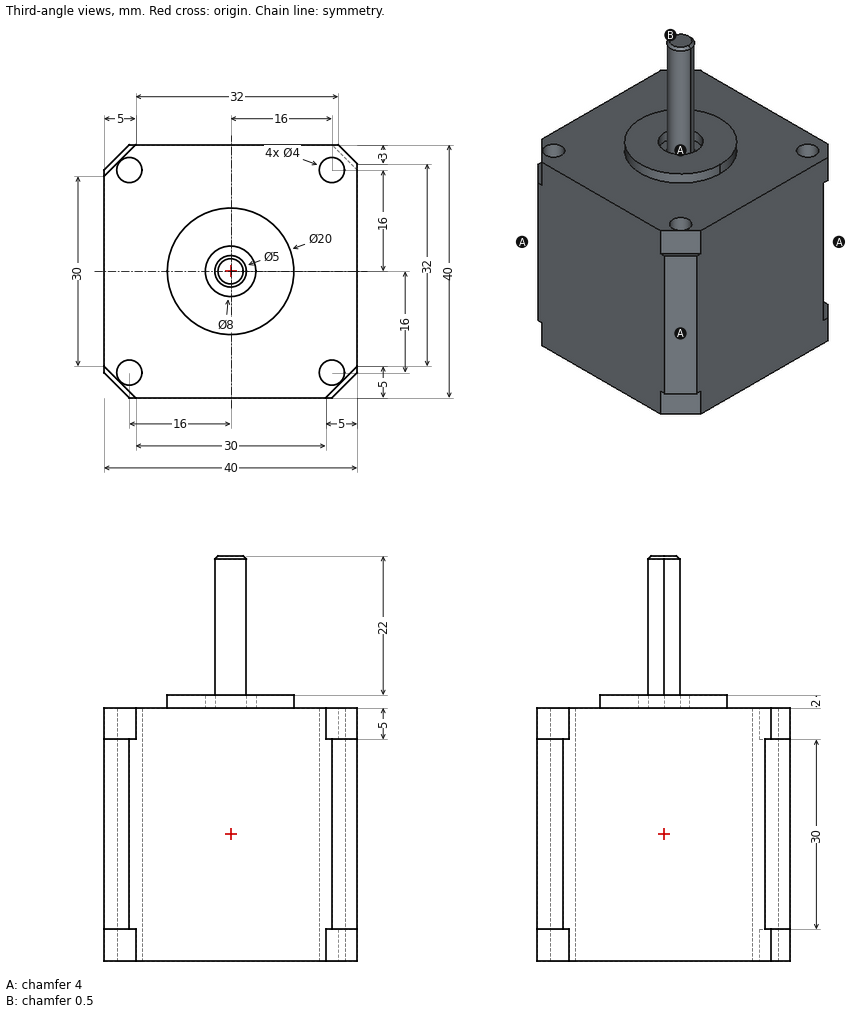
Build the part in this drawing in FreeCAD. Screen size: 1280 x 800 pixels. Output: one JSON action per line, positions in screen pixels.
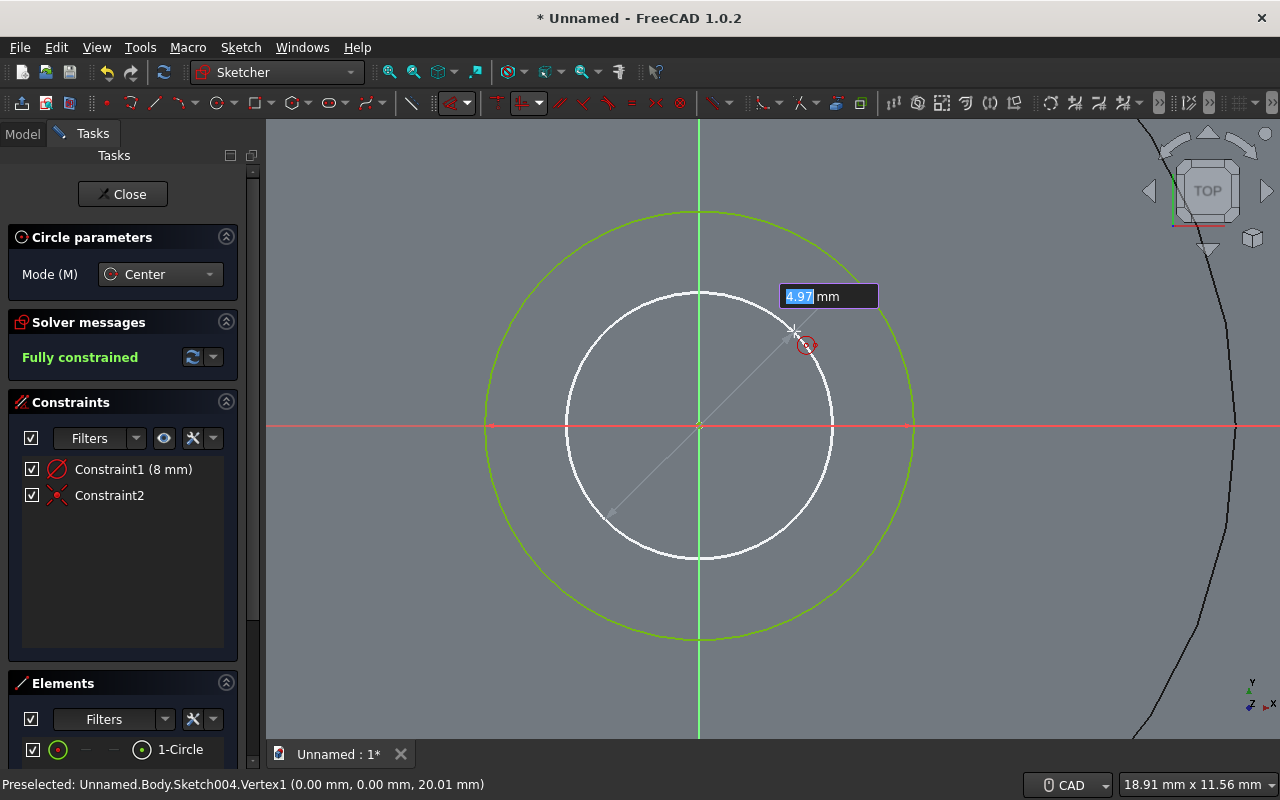
{"action": "type", "text": "5"}
{"action": "key", "text": "Return"}
{"action": "key", "text": "Escape"}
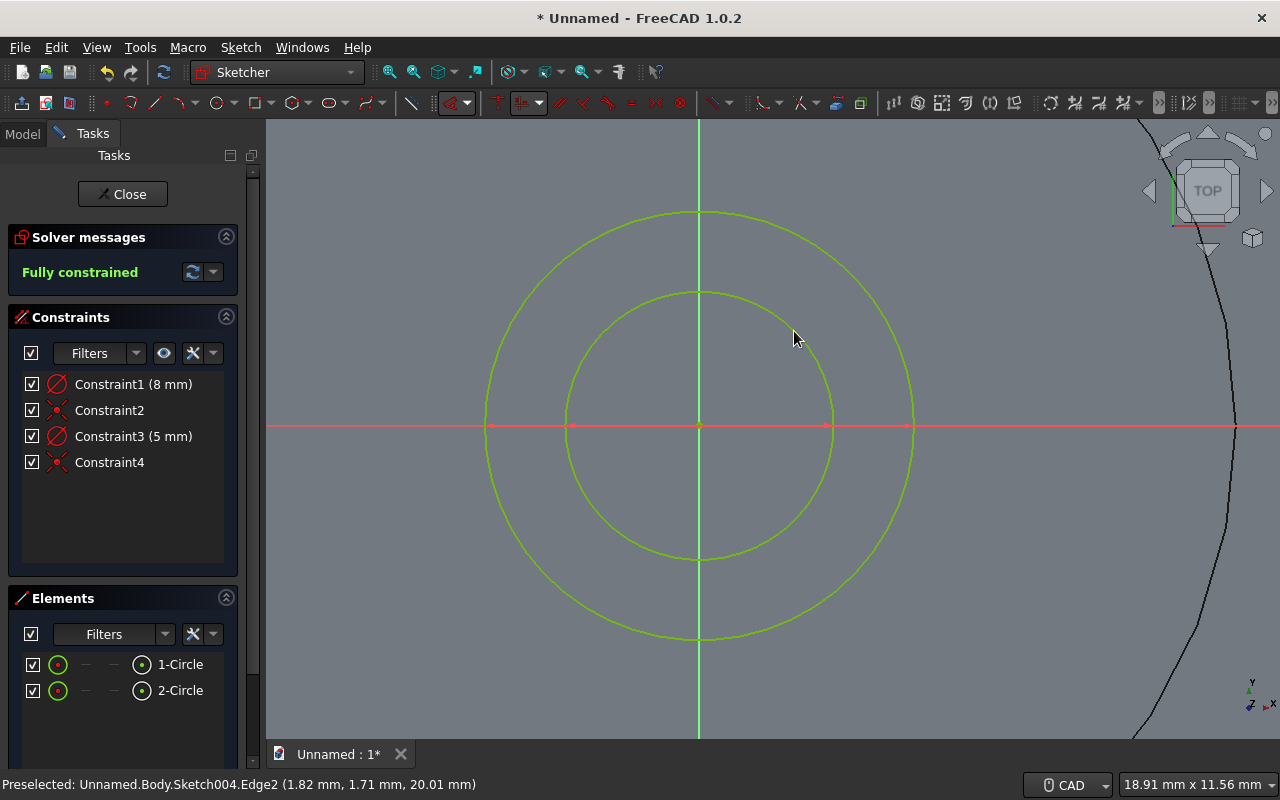
{"action": "left_click", "coordinate": [123, 194]}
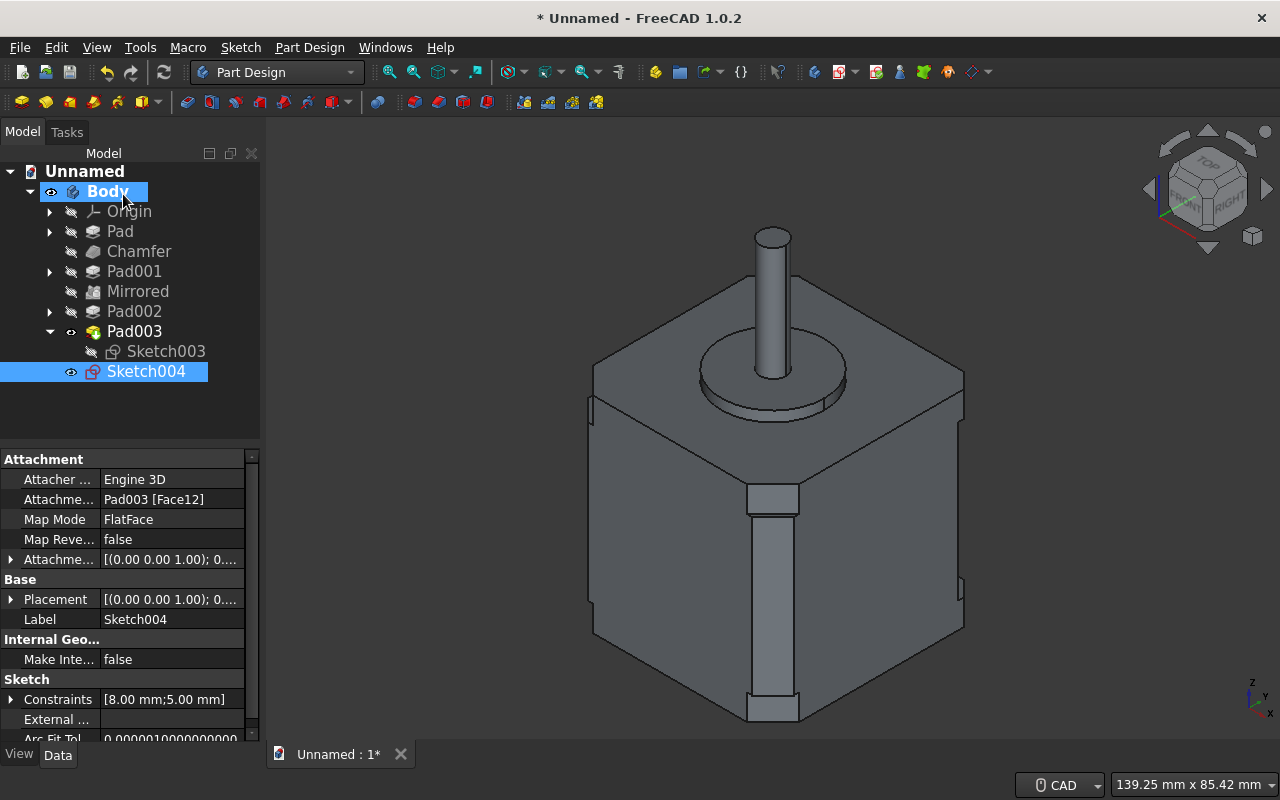
{"action": "left_click", "coordinate": [188, 102]}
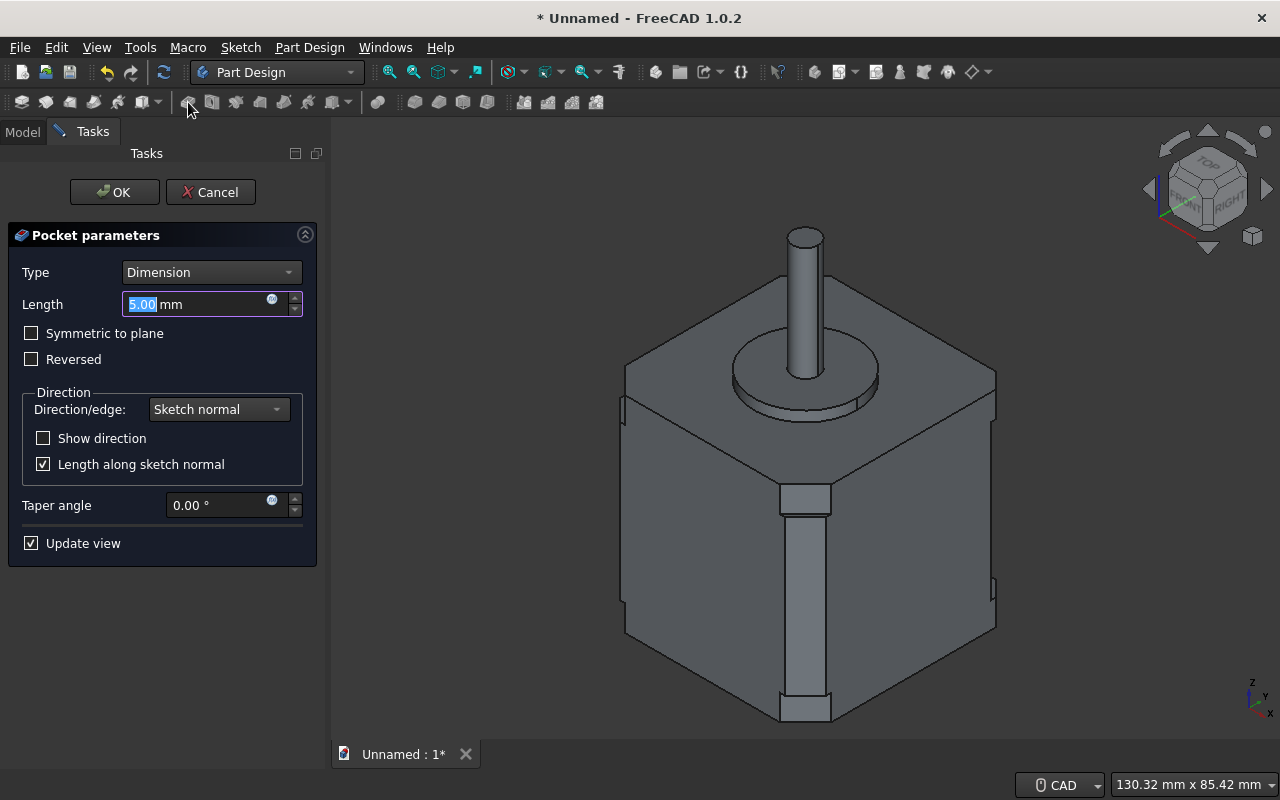
{"action": "type", "text": "2"}
{"action": "key", "text": "Tab"}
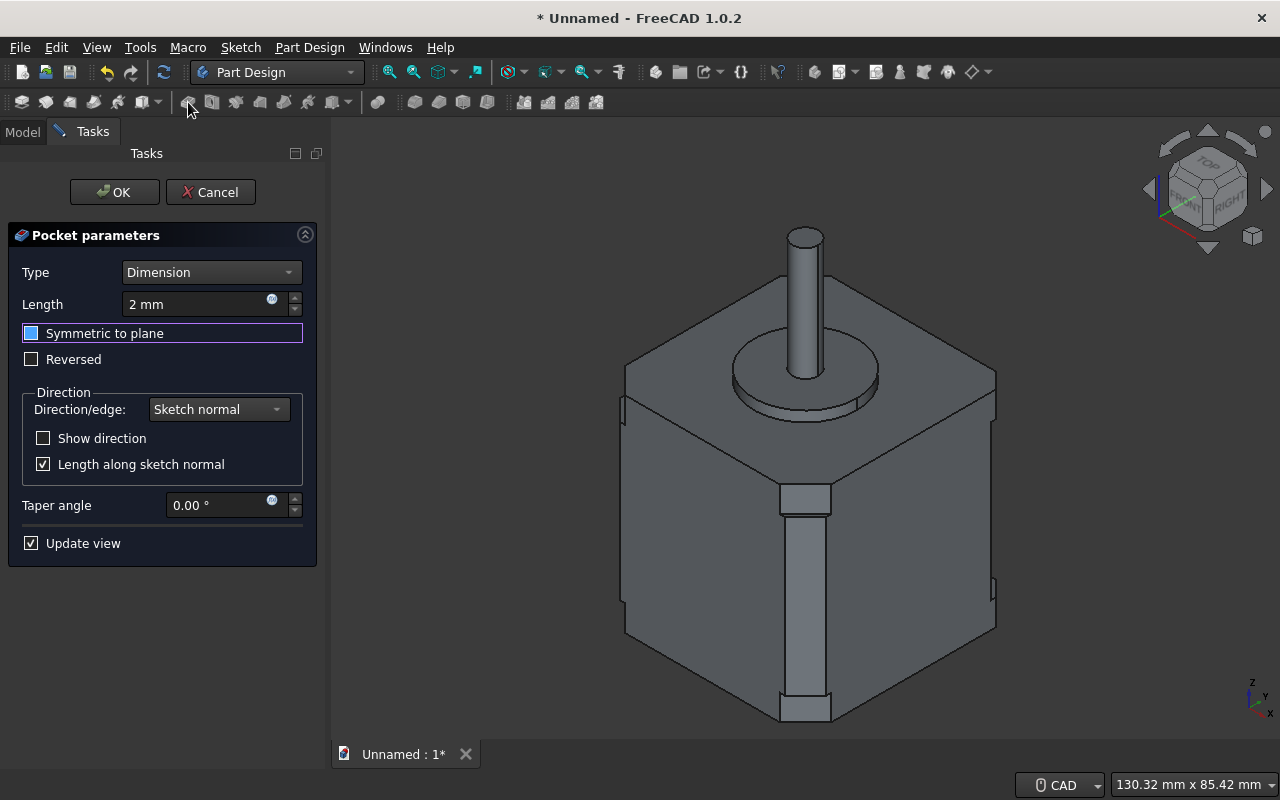
{"action": "left_click", "coordinate": [30, 359]}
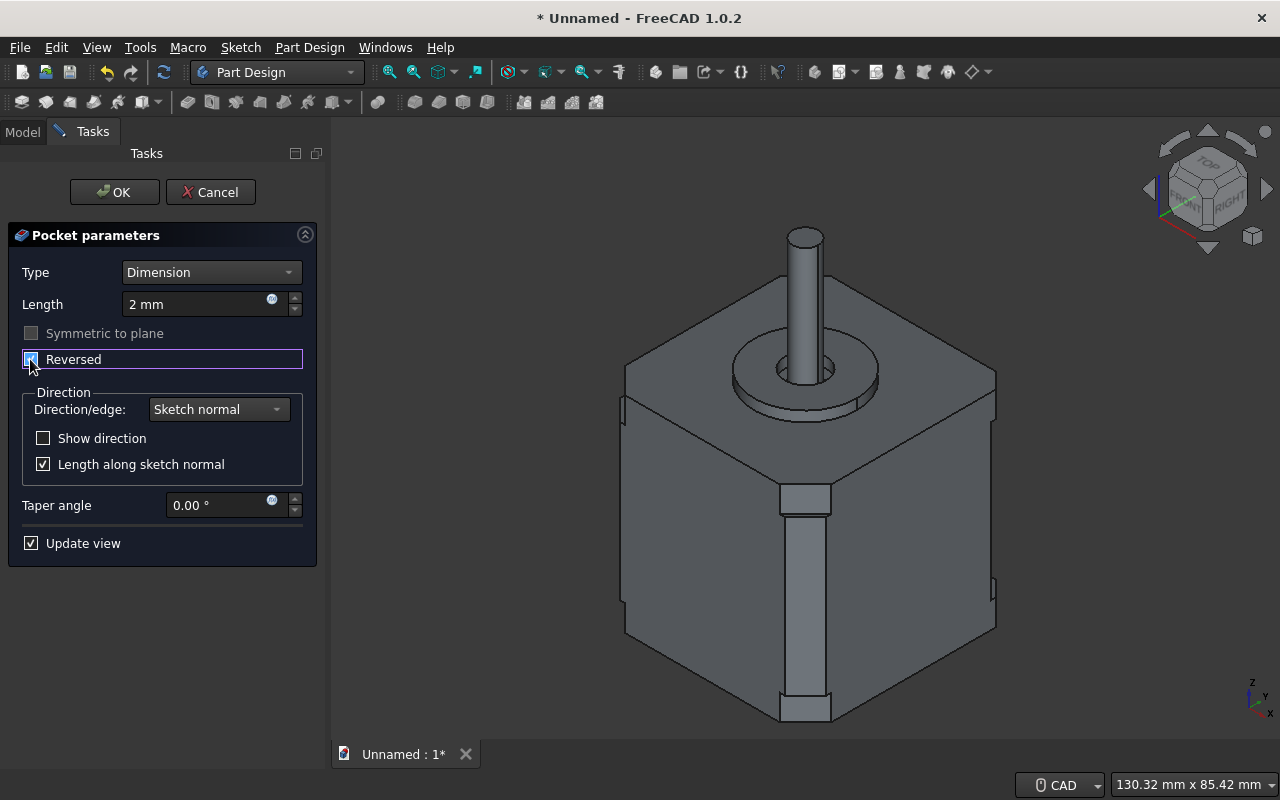
{"action": "left_click", "coordinate": [115, 192]}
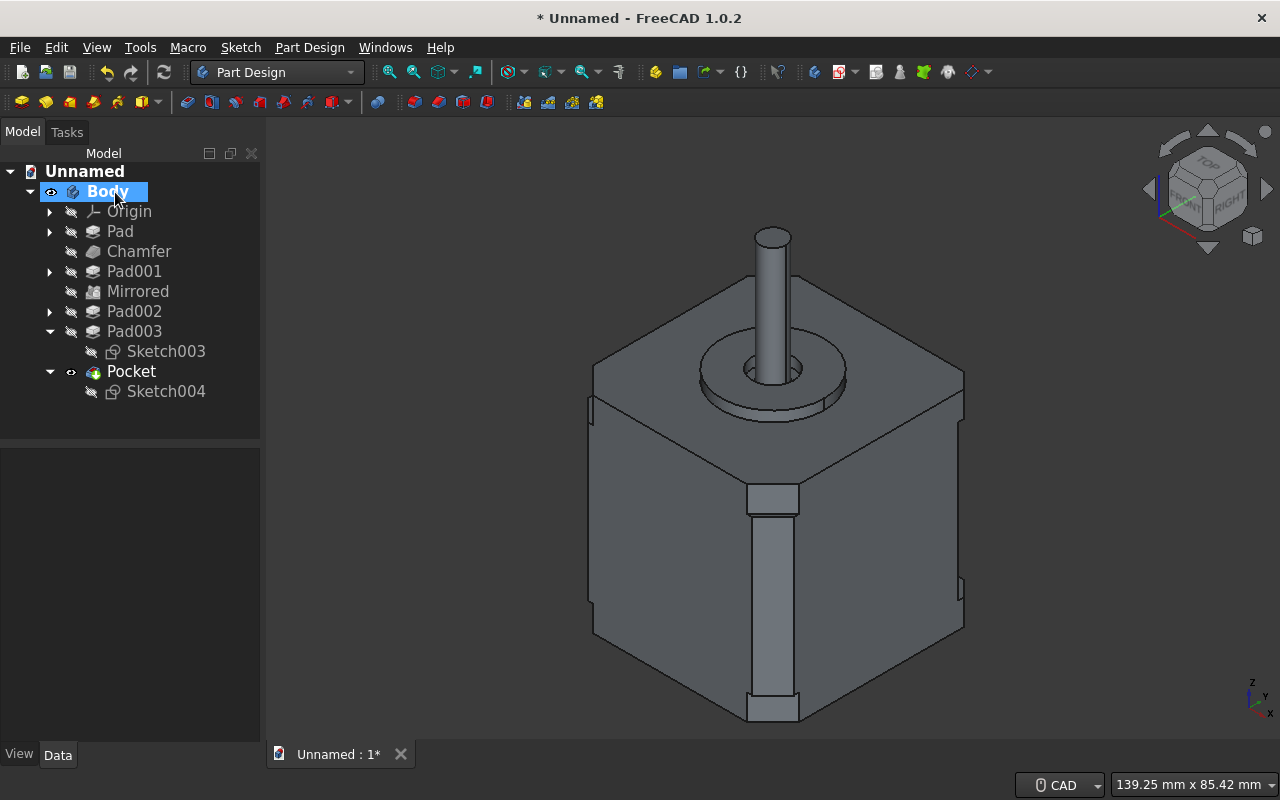
{"action": "left_click", "coordinate": [755, 235]}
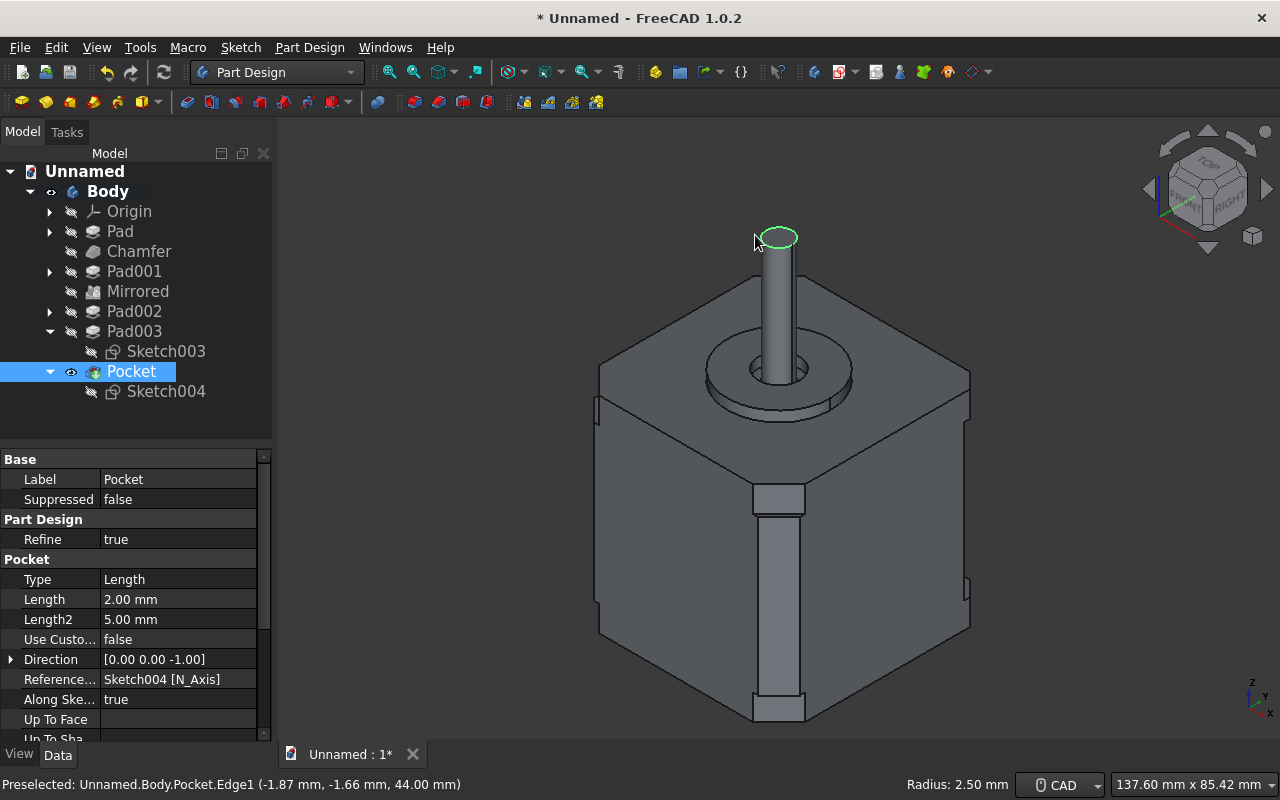
{"action": "left_click", "coordinate": [440, 102]}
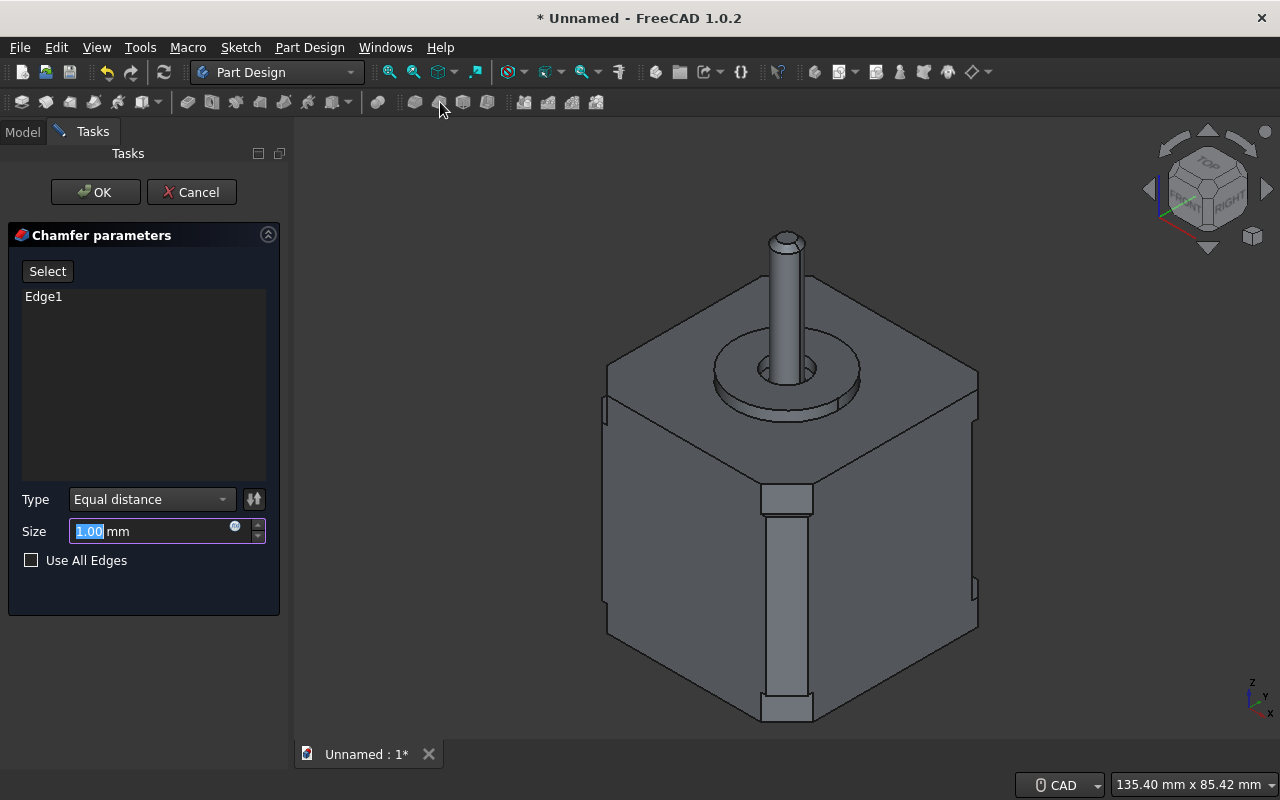
{"action": "type", "text": "0.5"}
{"action": "key", "text": "Tab"}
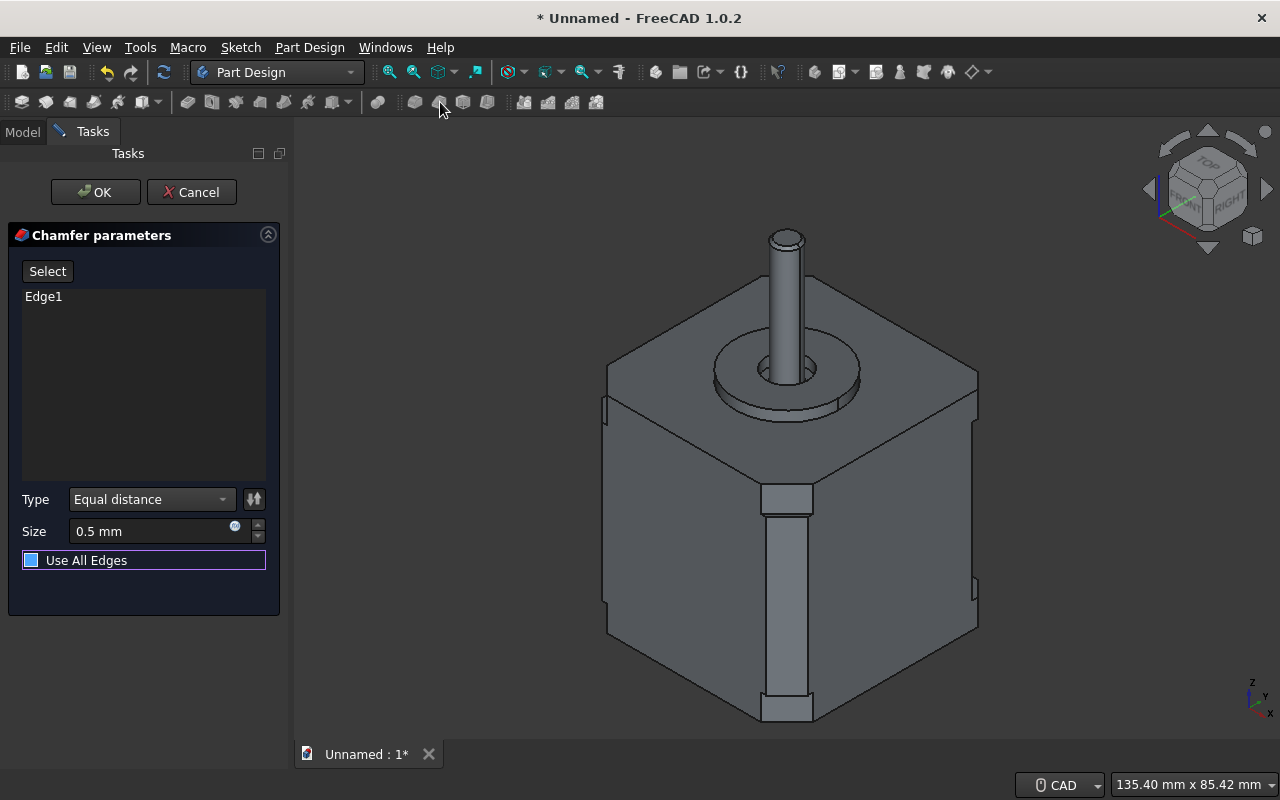
{"action": "left_click", "coordinate": [96, 192]}